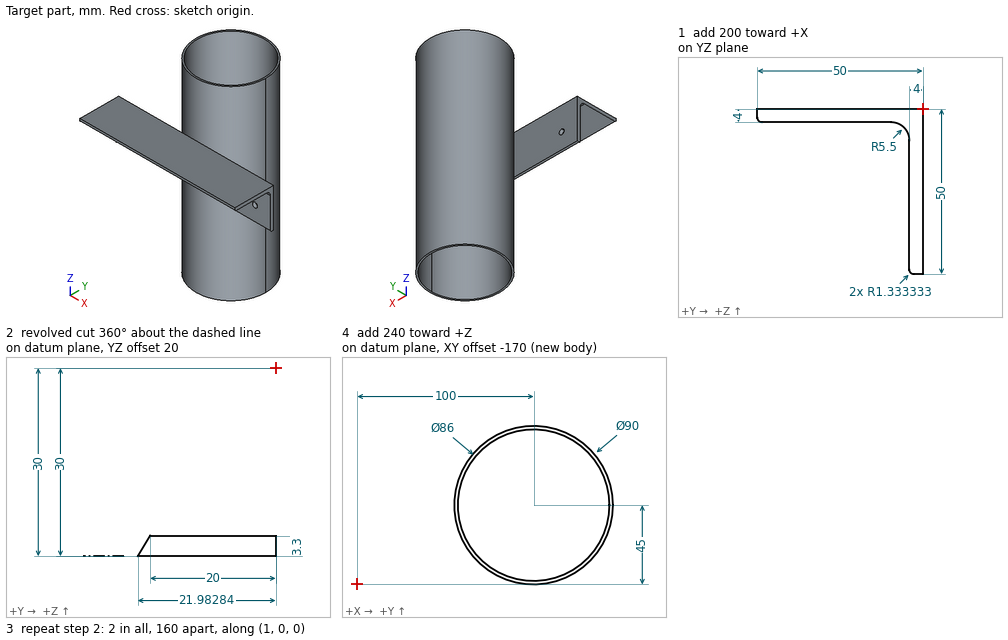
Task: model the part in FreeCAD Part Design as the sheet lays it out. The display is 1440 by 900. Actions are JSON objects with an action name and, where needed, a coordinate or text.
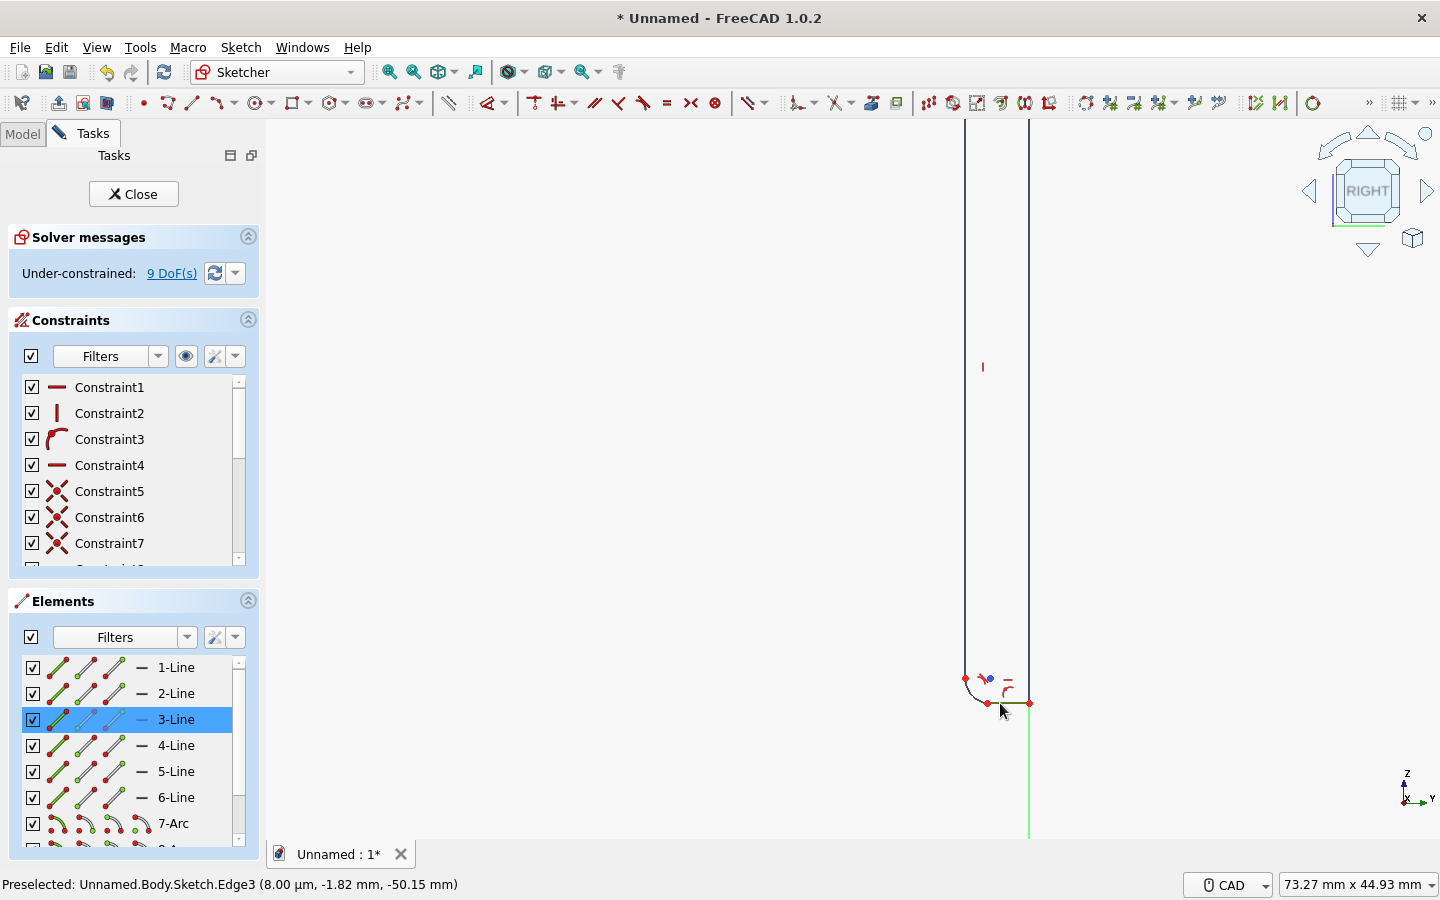
{"action": "scroll", "coordinate": [968, 689], "scroll_direction": "up", "scroll_amount": 2}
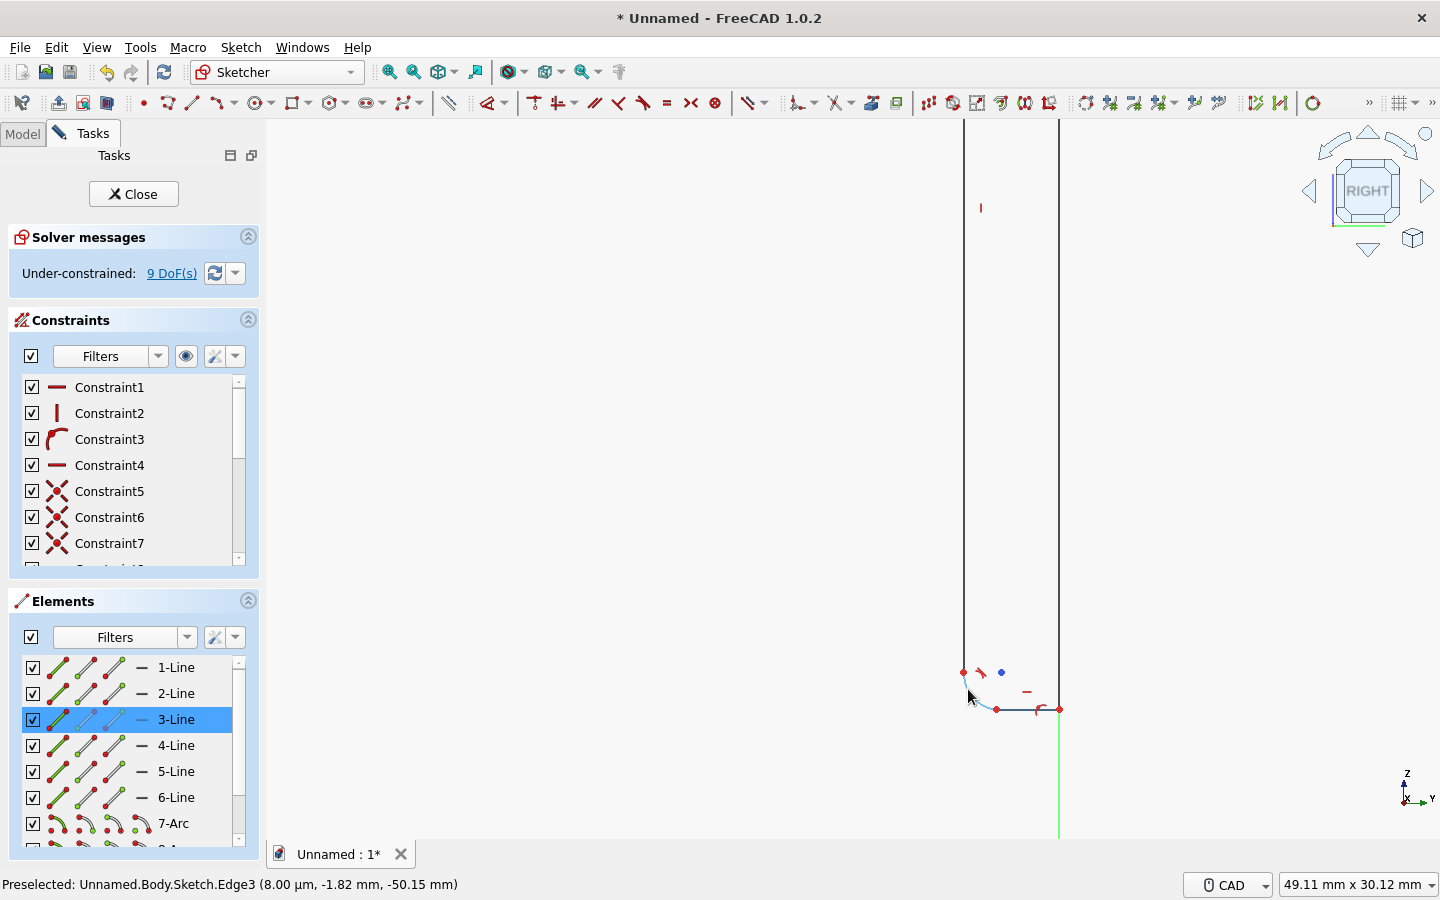
{"action": "left_click", "coordinate": [967, 689]}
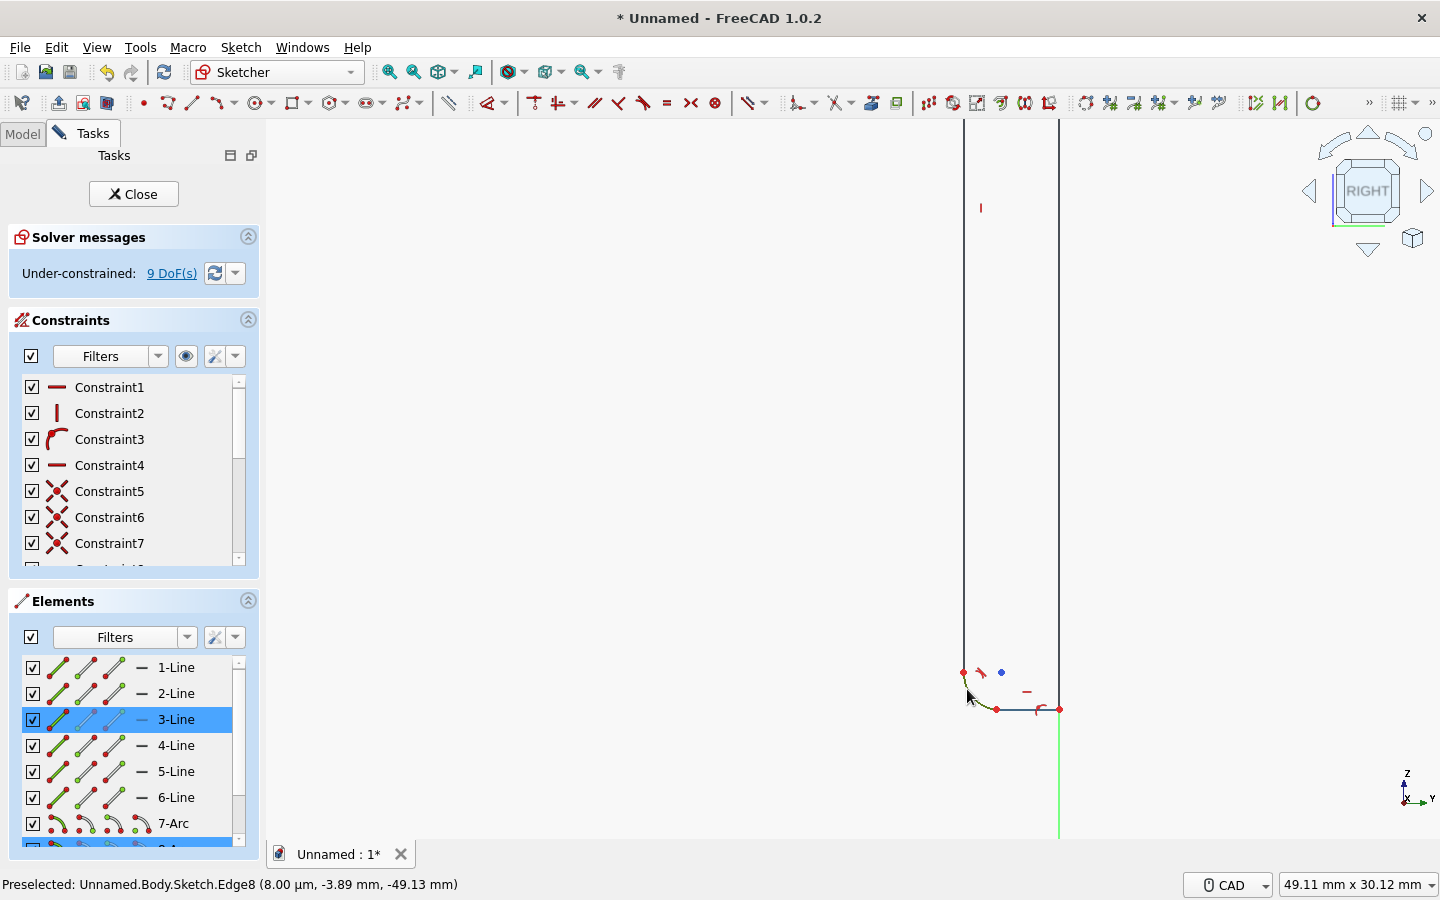
{"action": "left_click", "coordinate": [644, 104]}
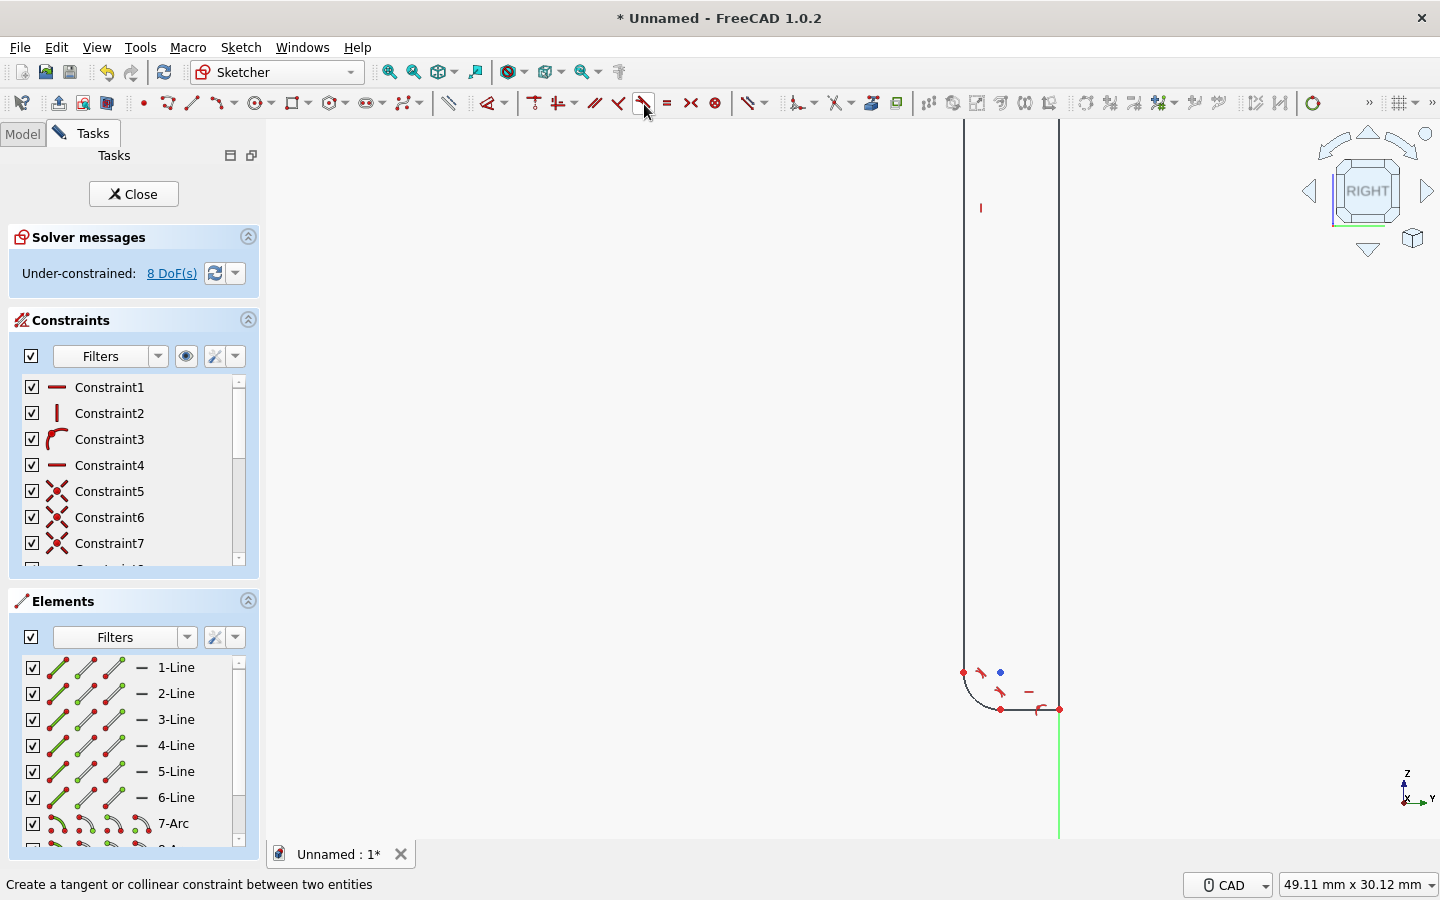
{"action": "scroll", "coordinate": [973, 694], "scroll_direction": "down", "scroll_amount": 5}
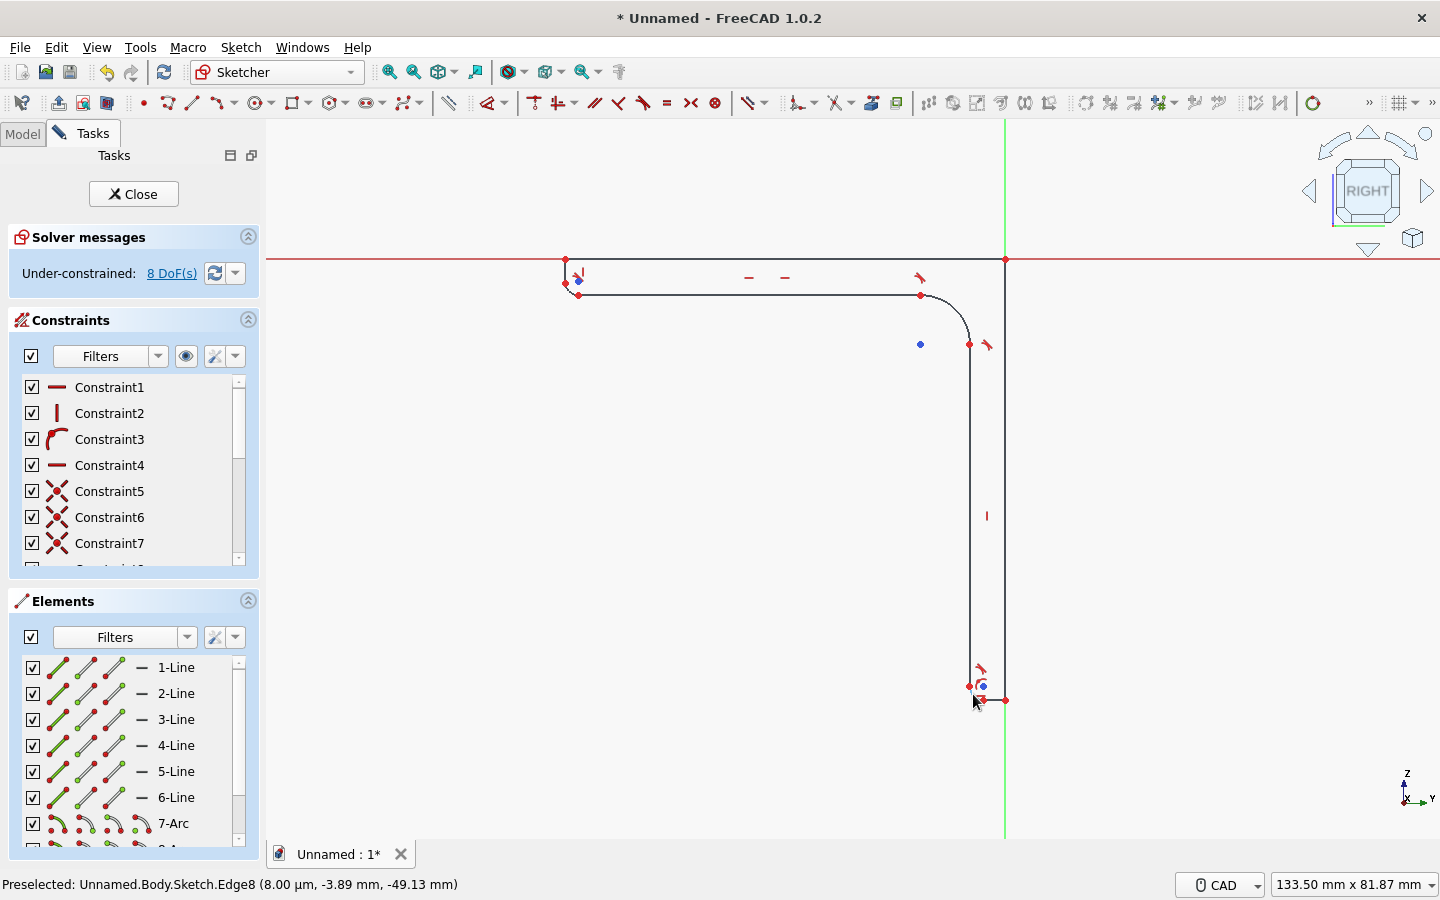
{"action": "scroll", "coordinate": [565, 267], "scroll_direction": "up", "scroll_amount": 4}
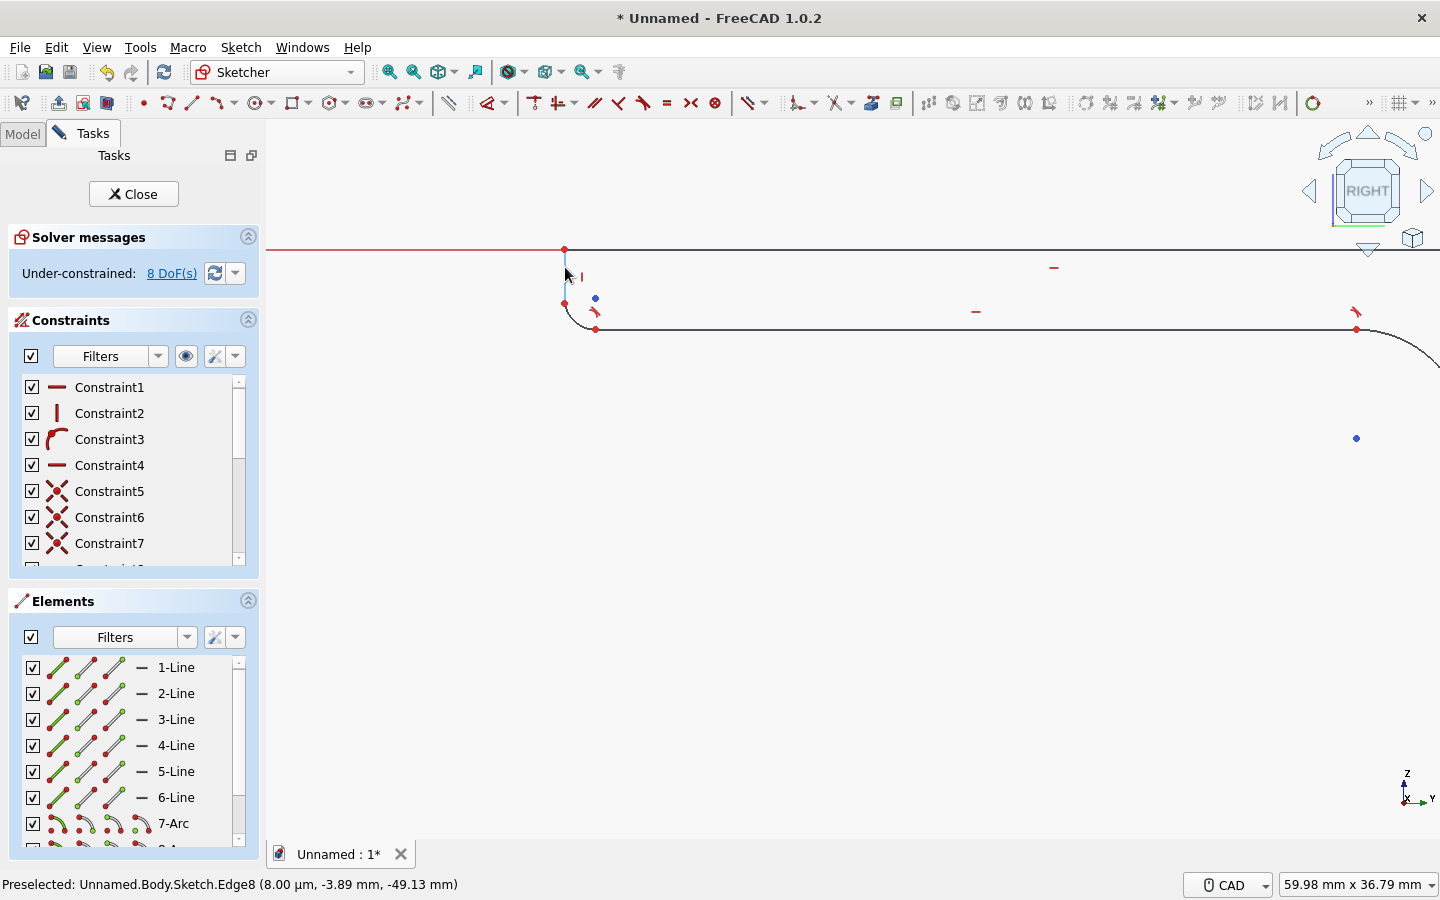
{"action": "left_click", "coordinate": [565, 266]}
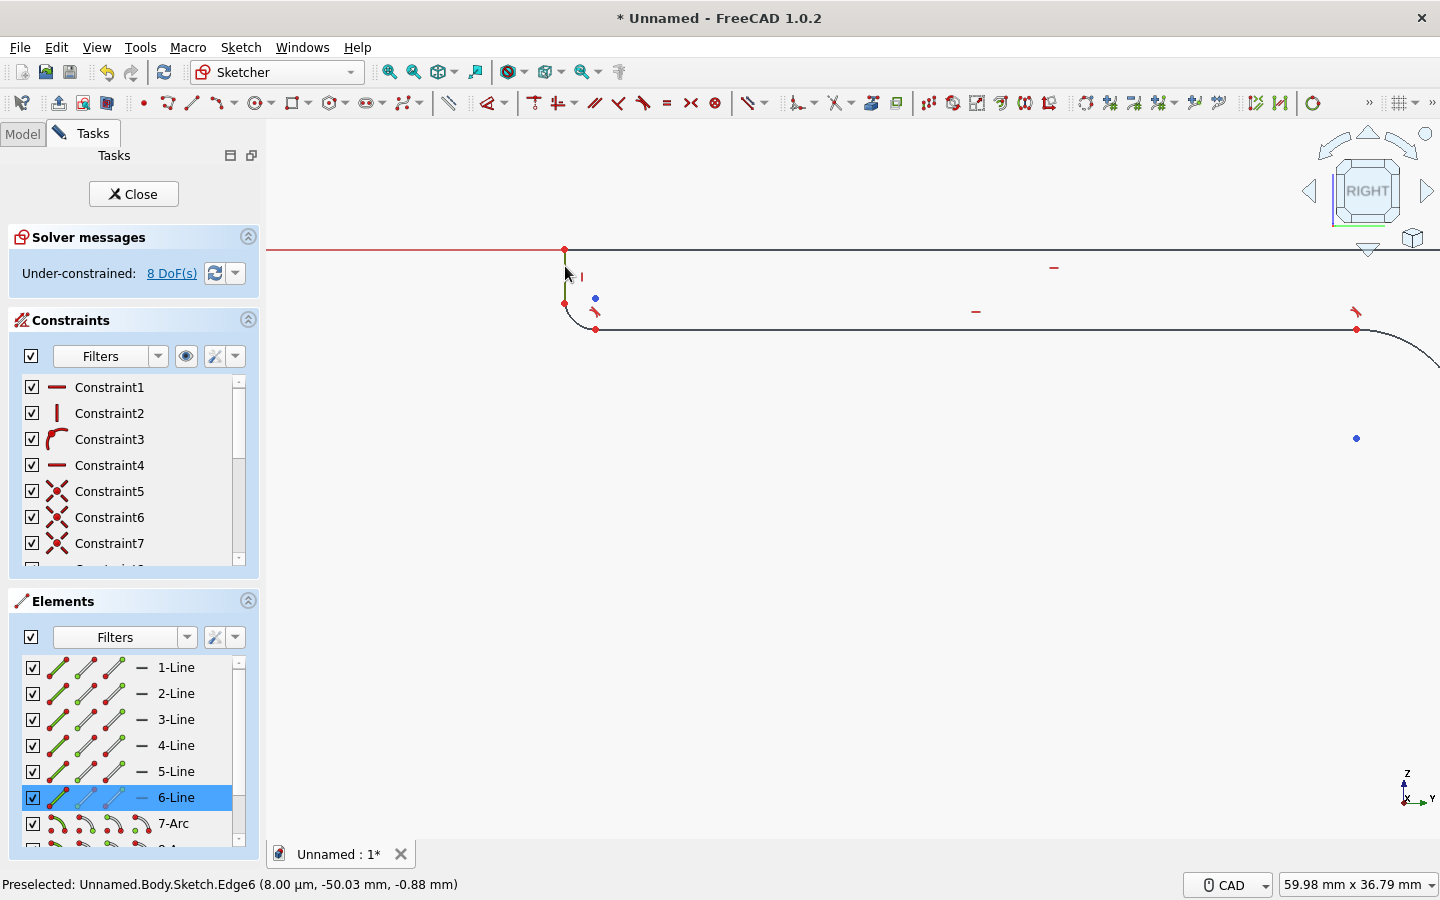
{"action": "left_click", "coordinate": [570, 316]}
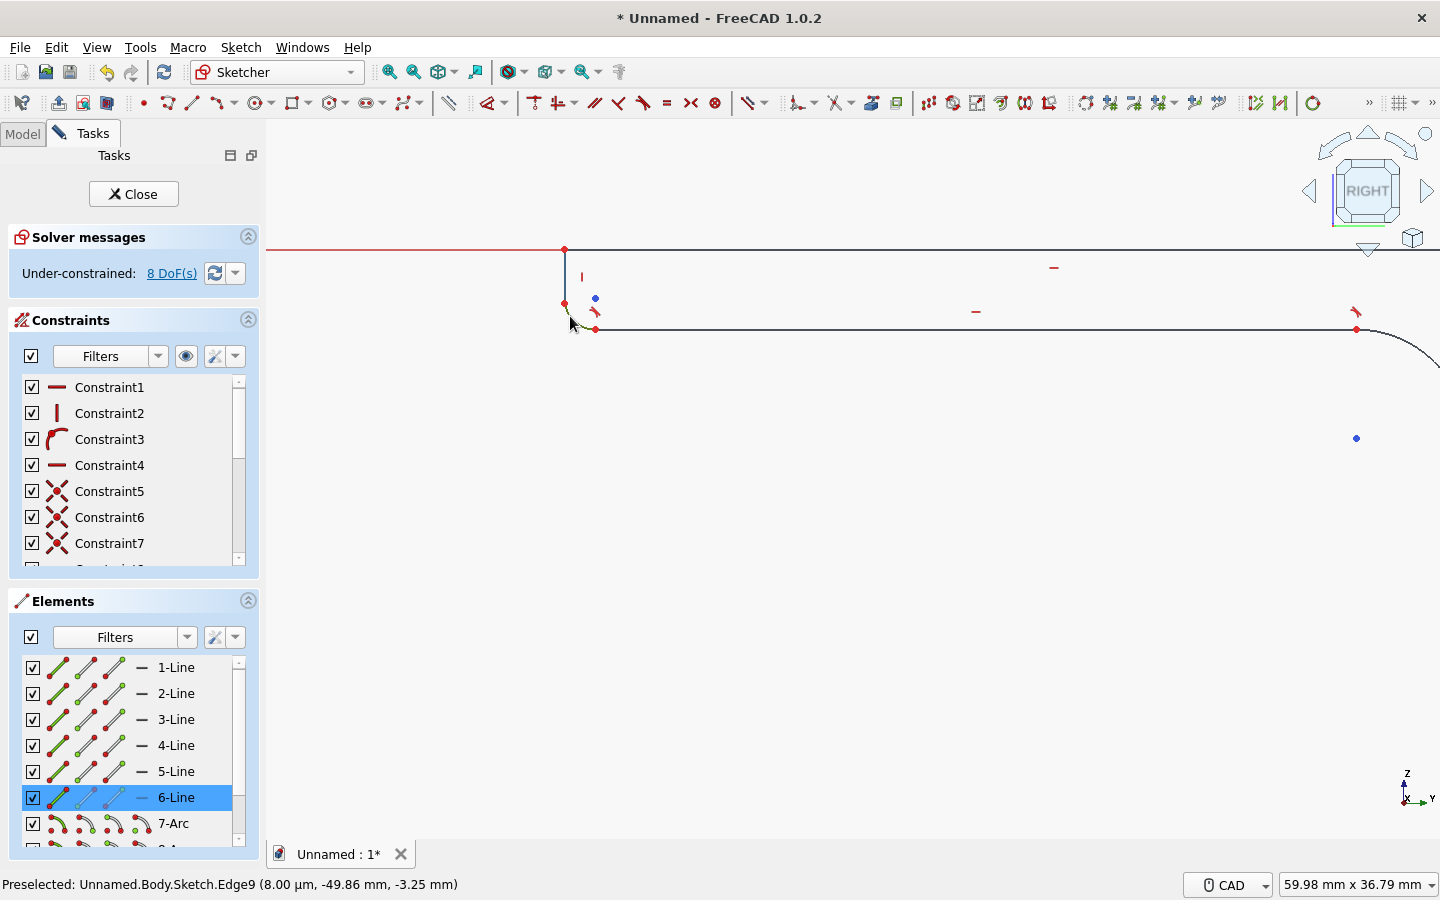
{"action": "left_click", "coordinate": [644, 104]}